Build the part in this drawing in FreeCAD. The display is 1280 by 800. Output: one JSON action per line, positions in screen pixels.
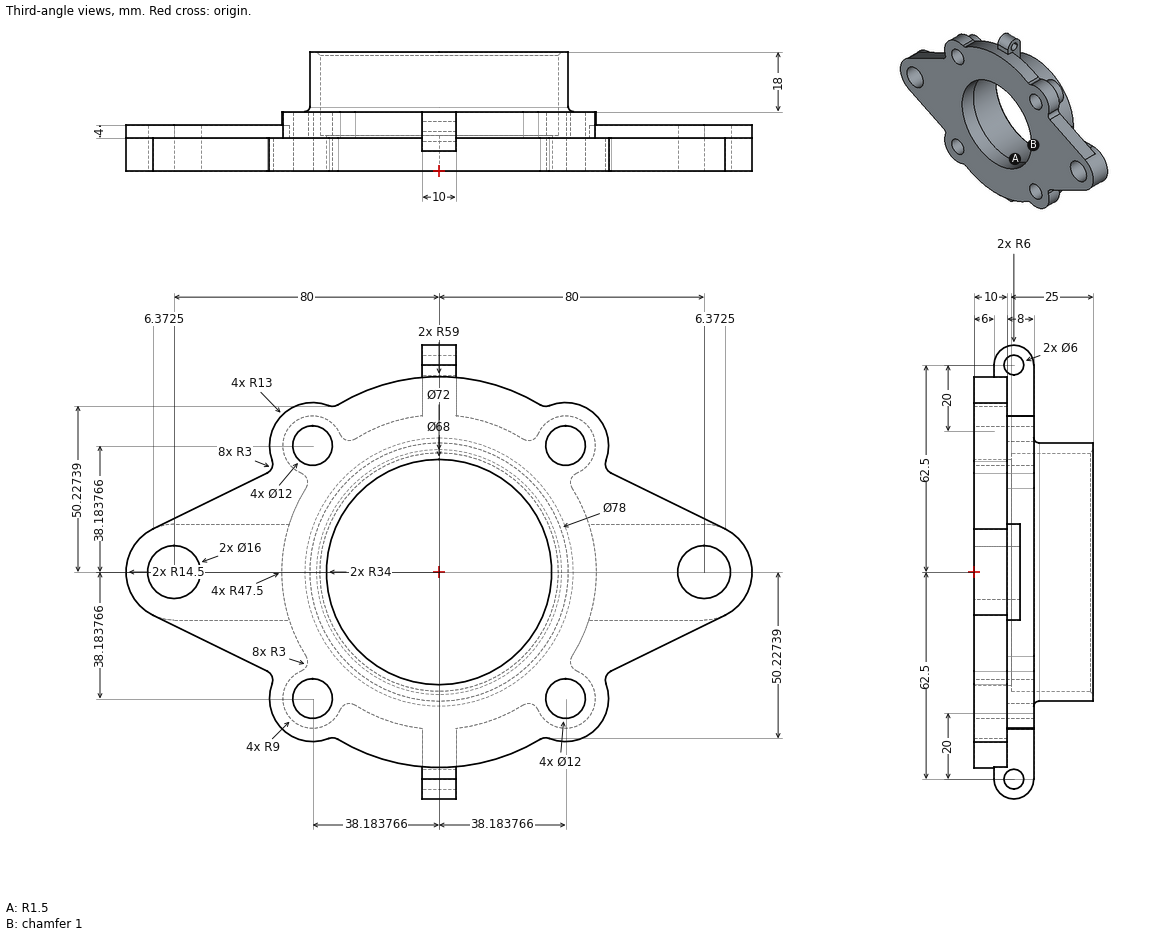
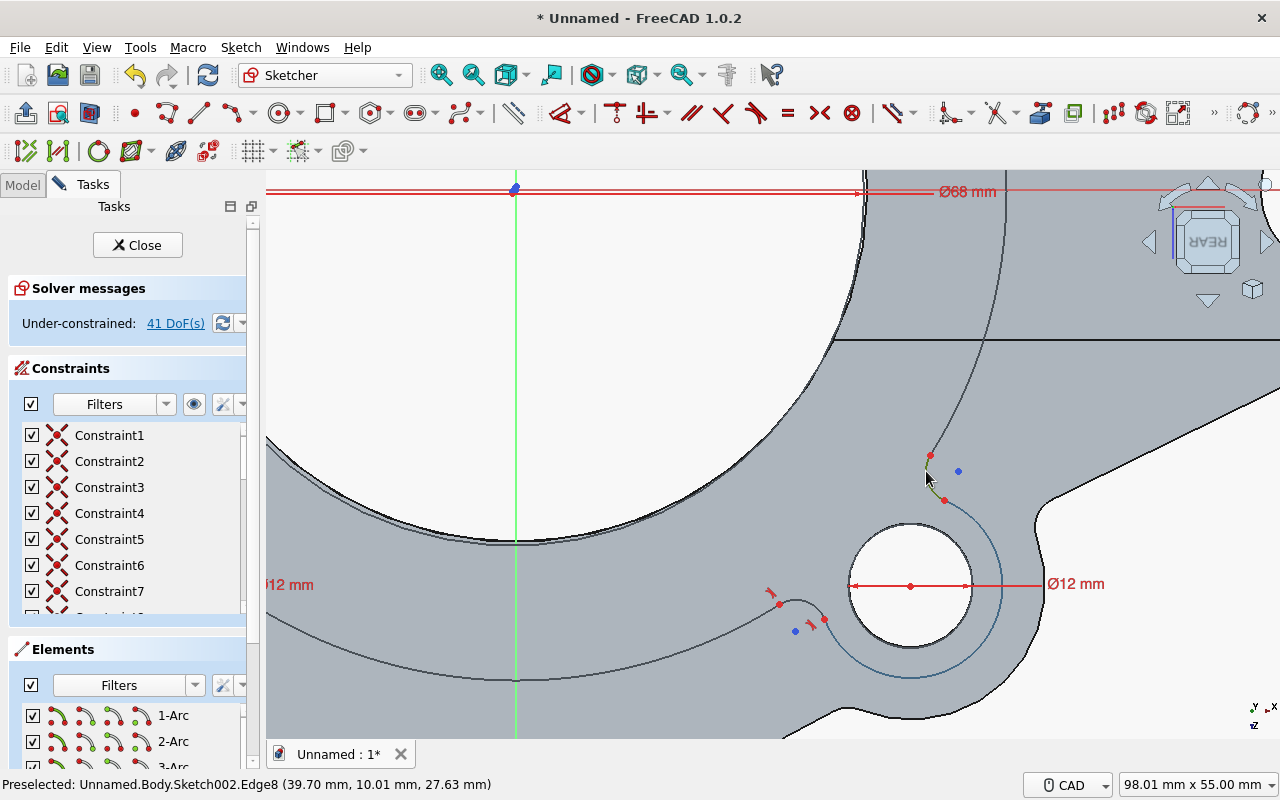
{"action": "left_click", "coordinate": [756, 114]}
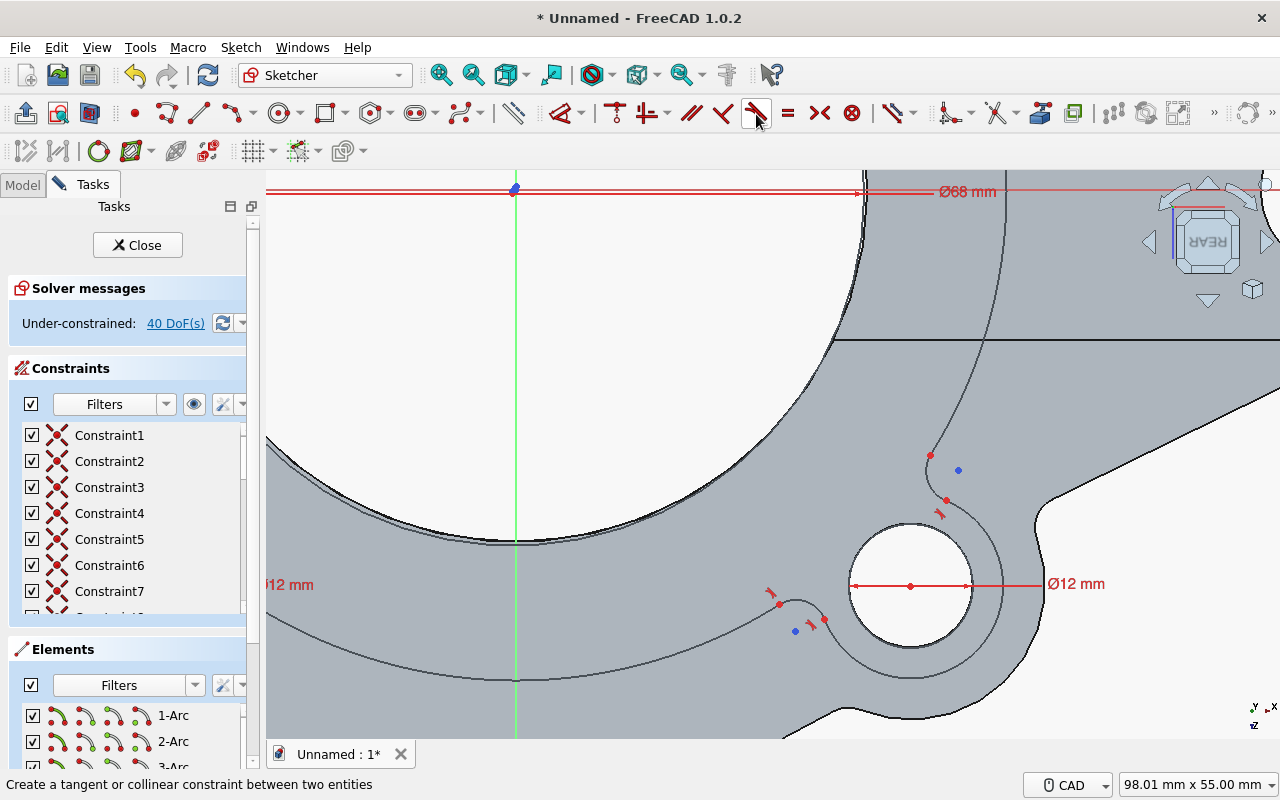
{"action": "left_click", "coordinate": [926, 471]}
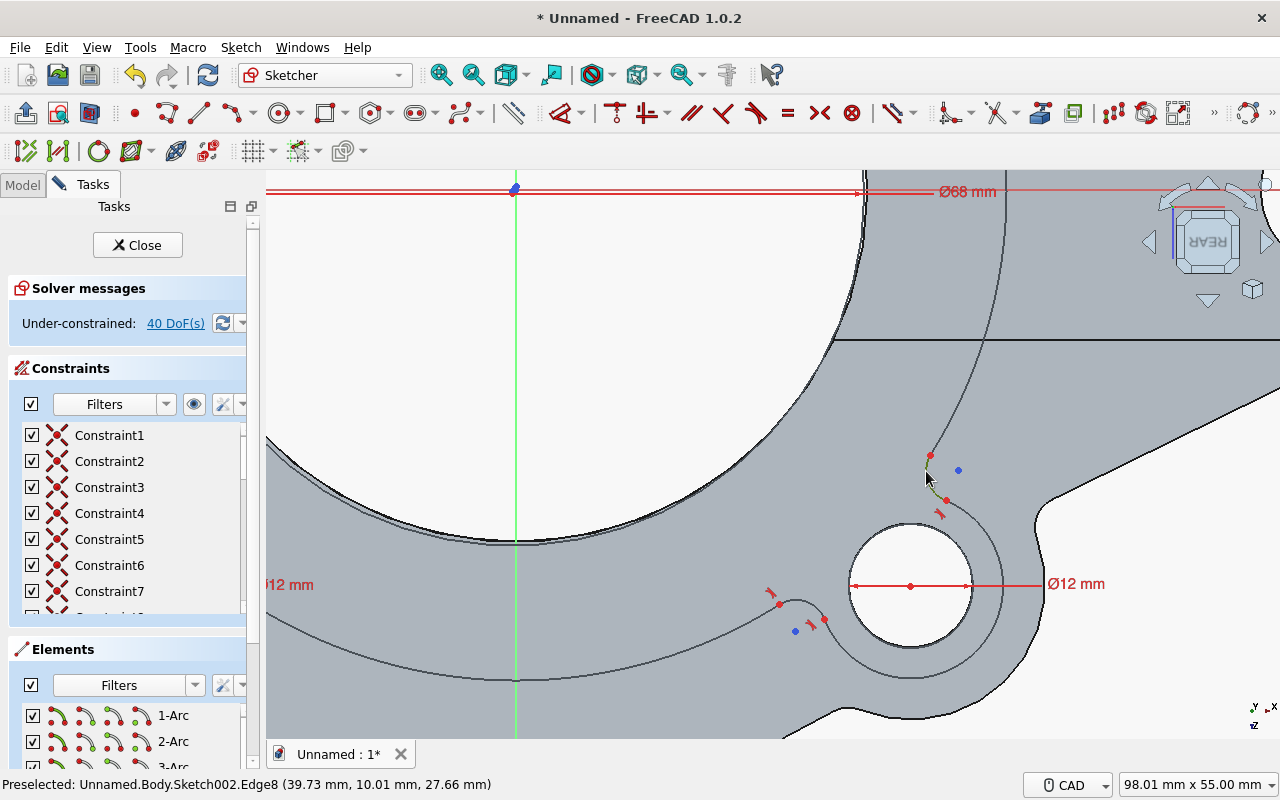
{"action": "left_click", "coordinate": [994, 302]}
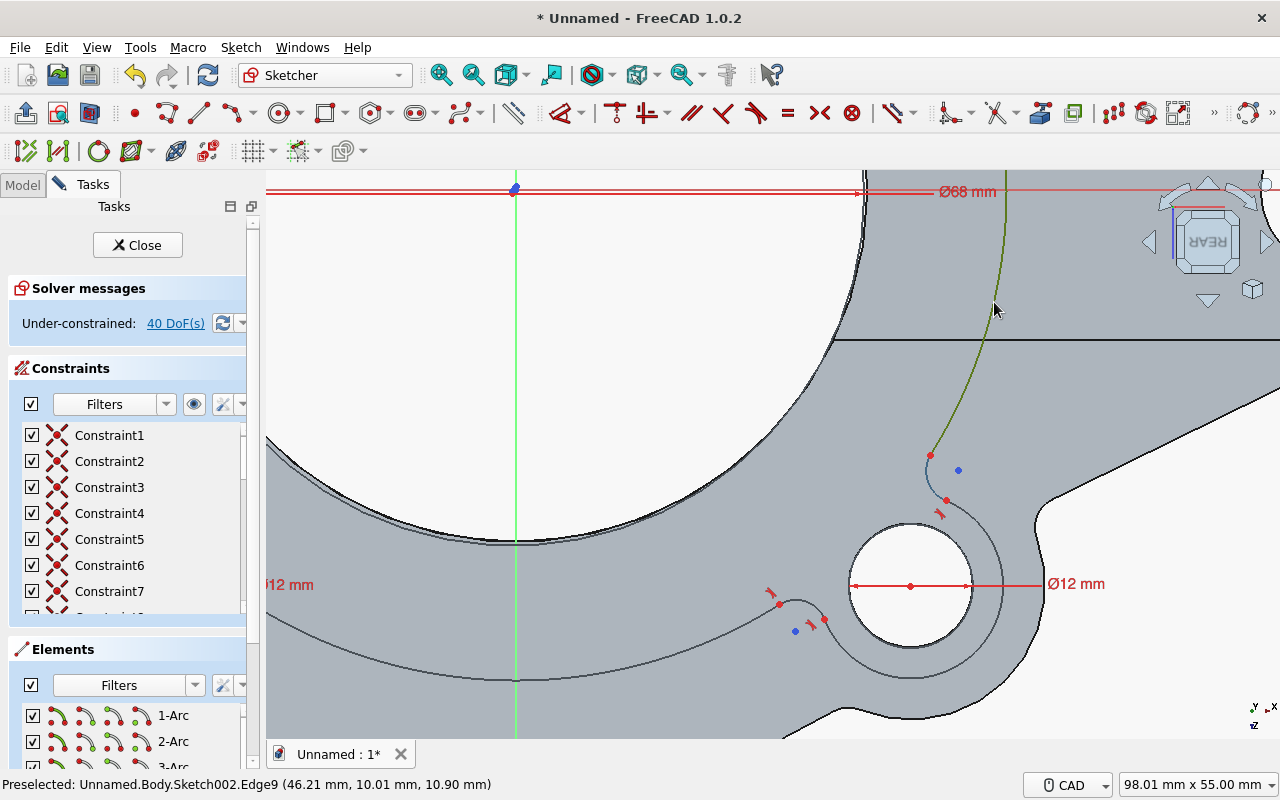
{"action": "left_click", "coordinate": [756, 114]}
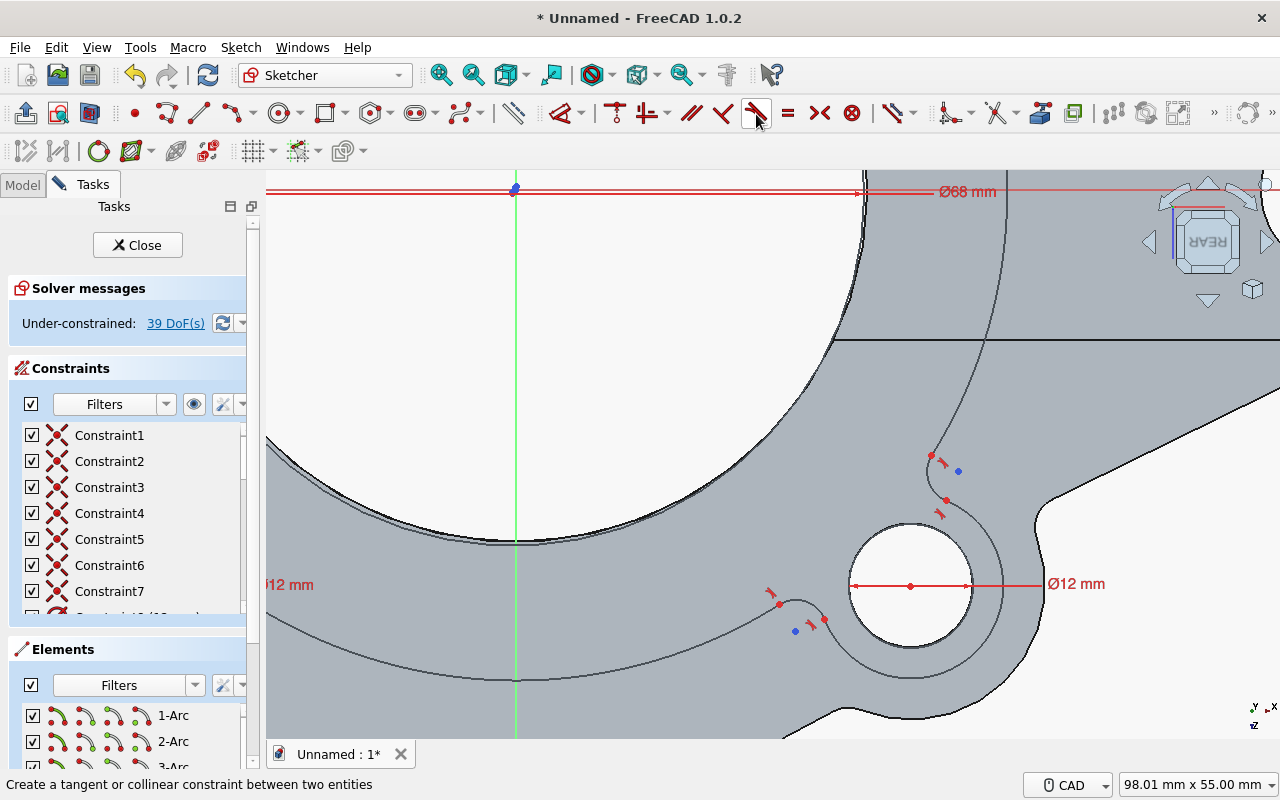
{"action": "left_click", "coordinate": [995, 302]}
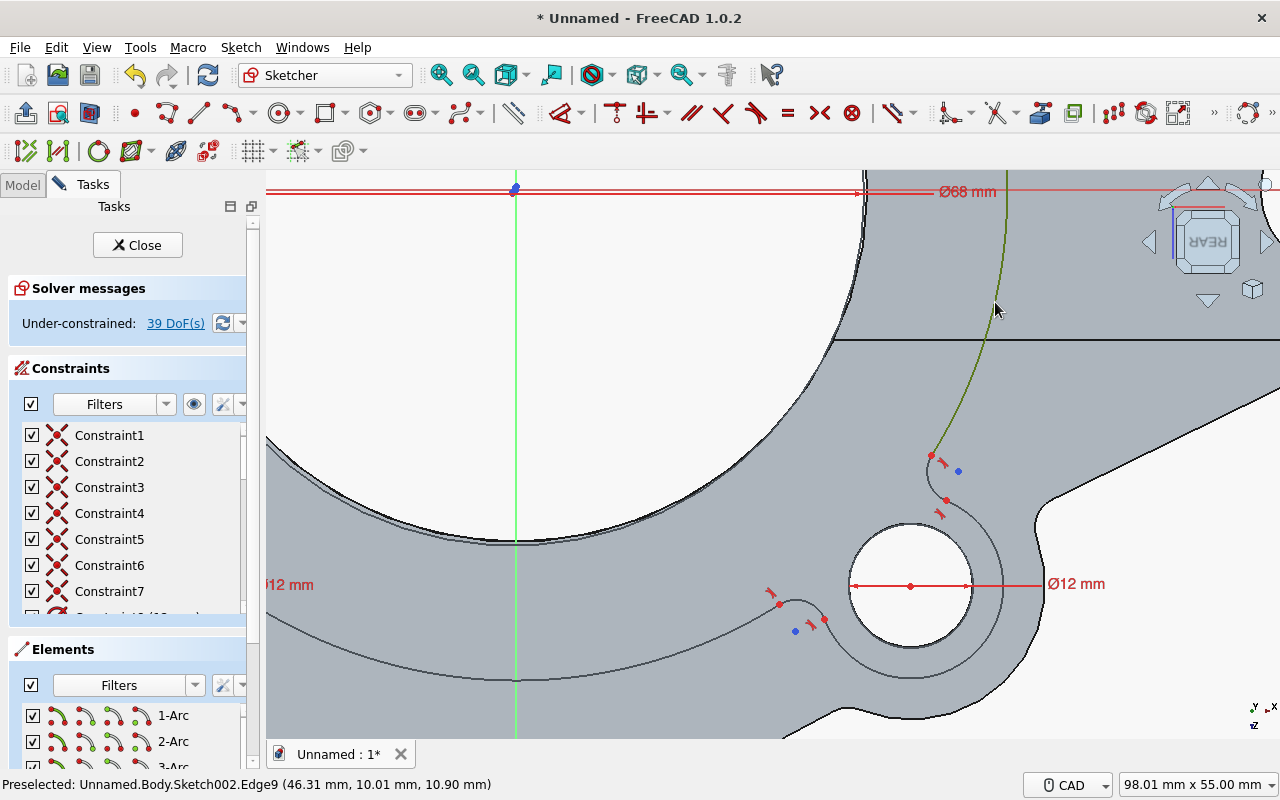
{"action": "scroll", "coordinate": [814, 608], "scroll_direction": "down", "scroll_amount": 5}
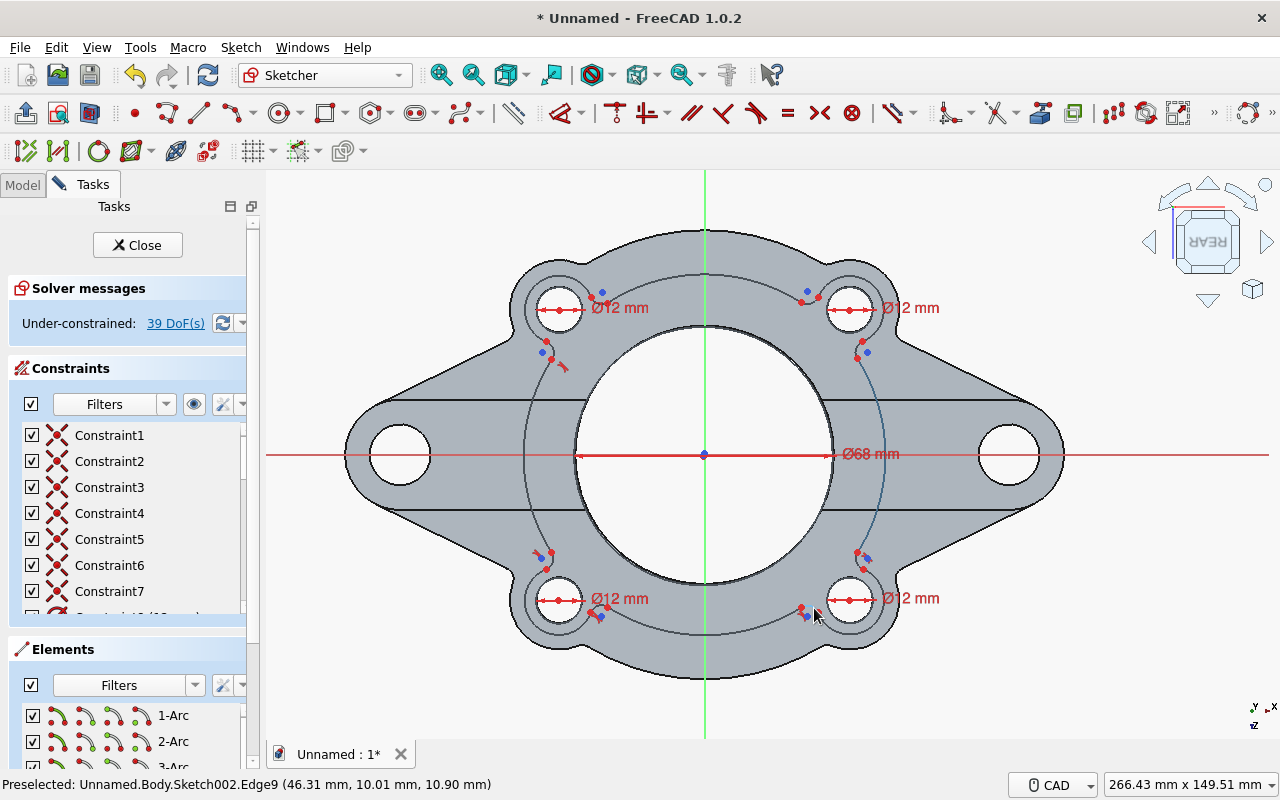
{"action": "scroll", "coordinate": [858, 345], "scroll_direction": "up", "scroll_amount": 5}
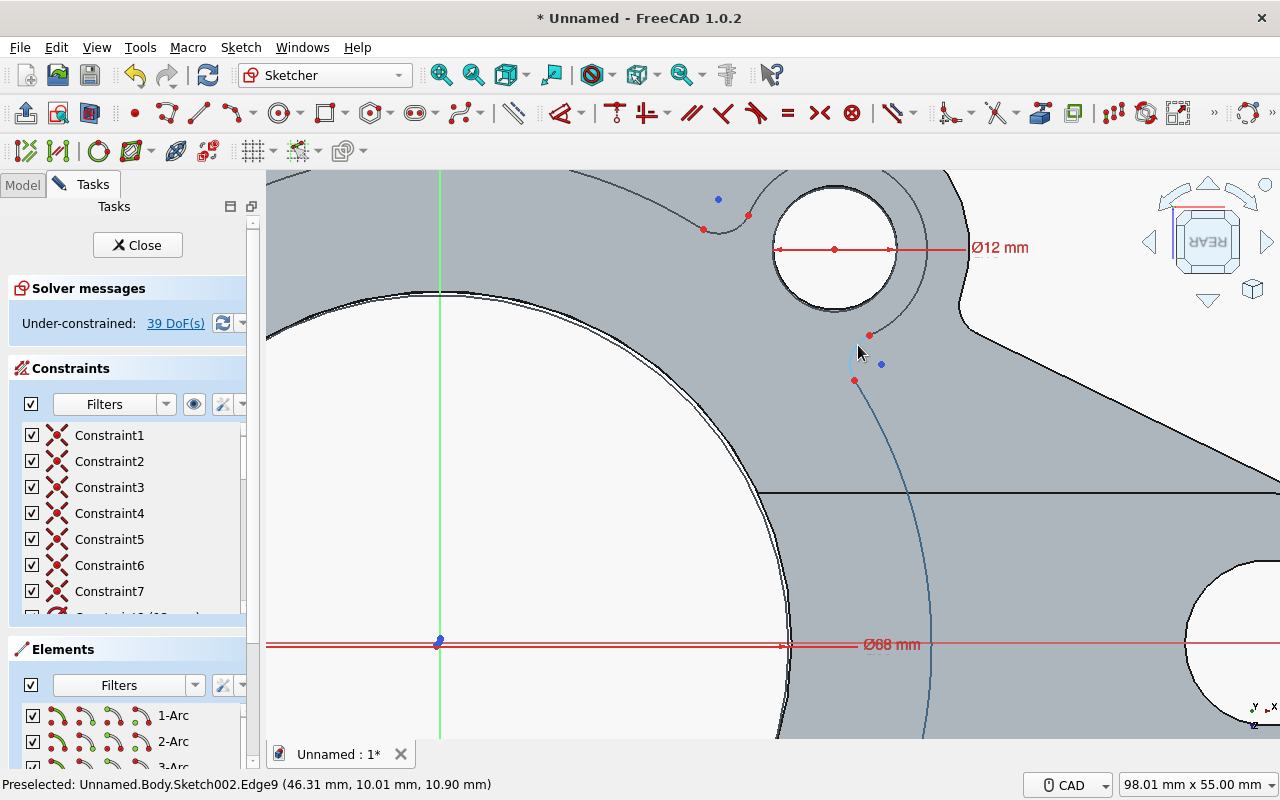
{"action": "left_click", "coordinate": [857, 345]}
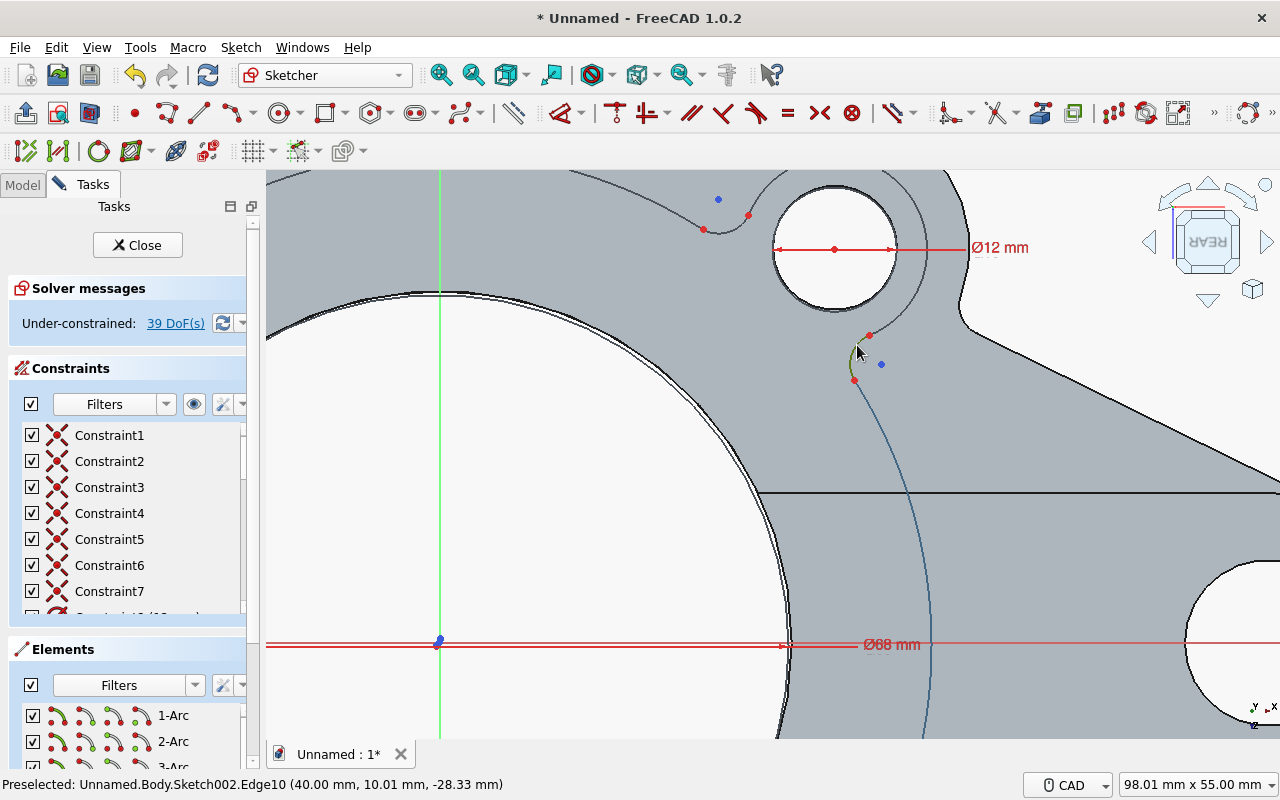
{"action": "left_click", "coordinate": [756, 114]}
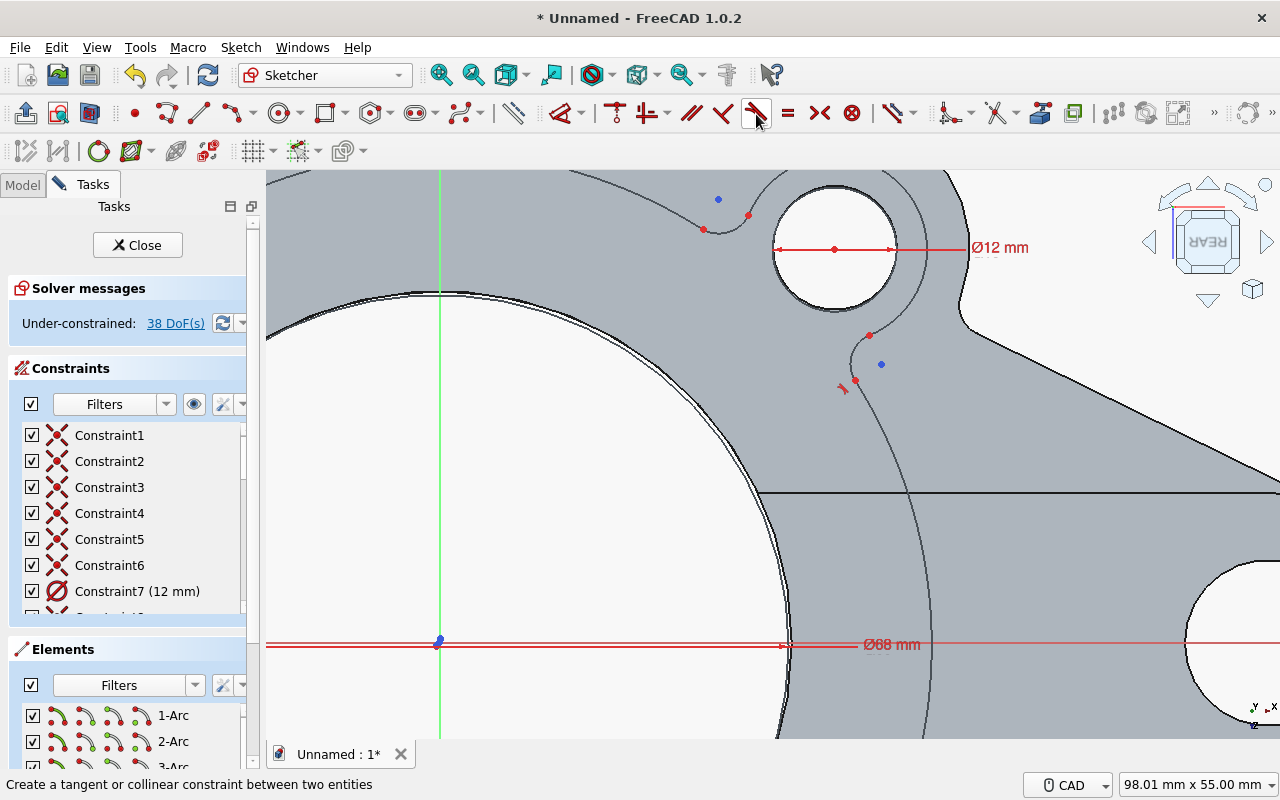
{"action": "left_click", "coordinate": [857, 345]}